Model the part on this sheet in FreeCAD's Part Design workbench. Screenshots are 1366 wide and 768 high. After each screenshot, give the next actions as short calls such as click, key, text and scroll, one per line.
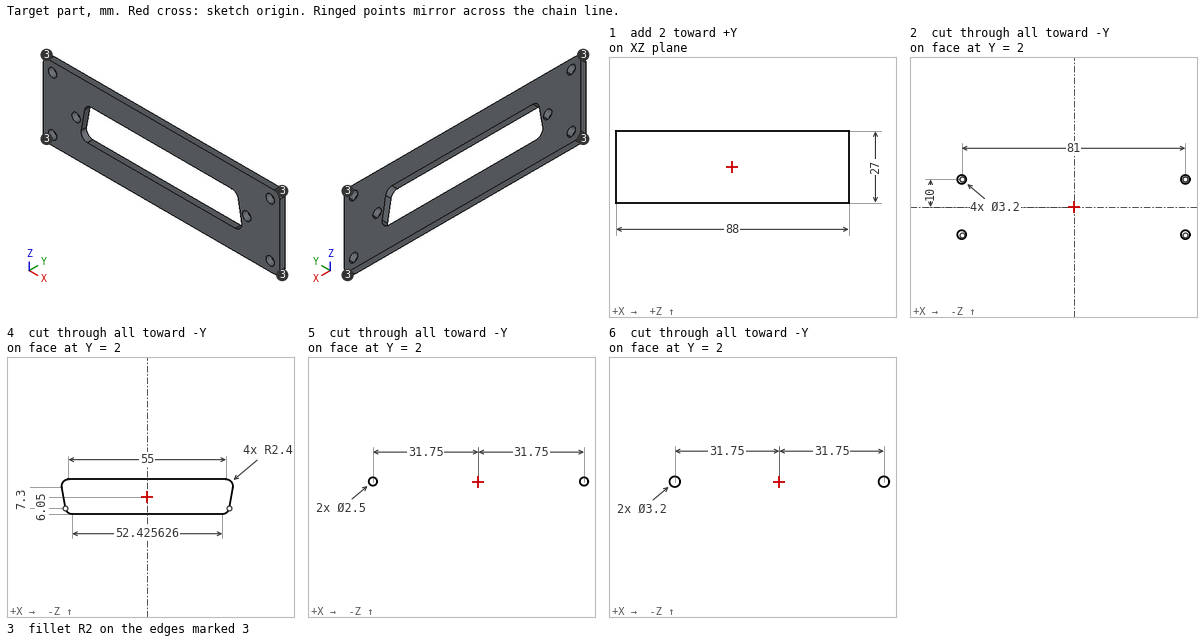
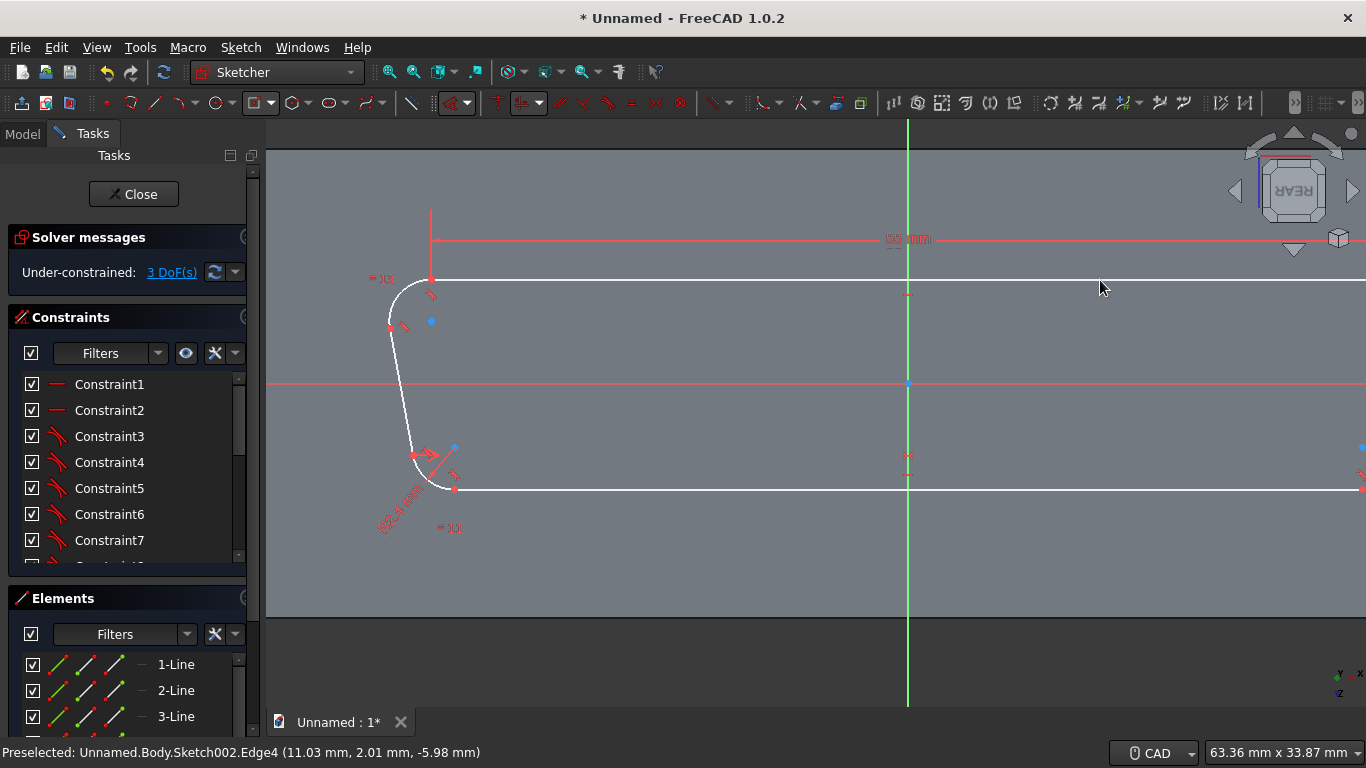
click(397, 367)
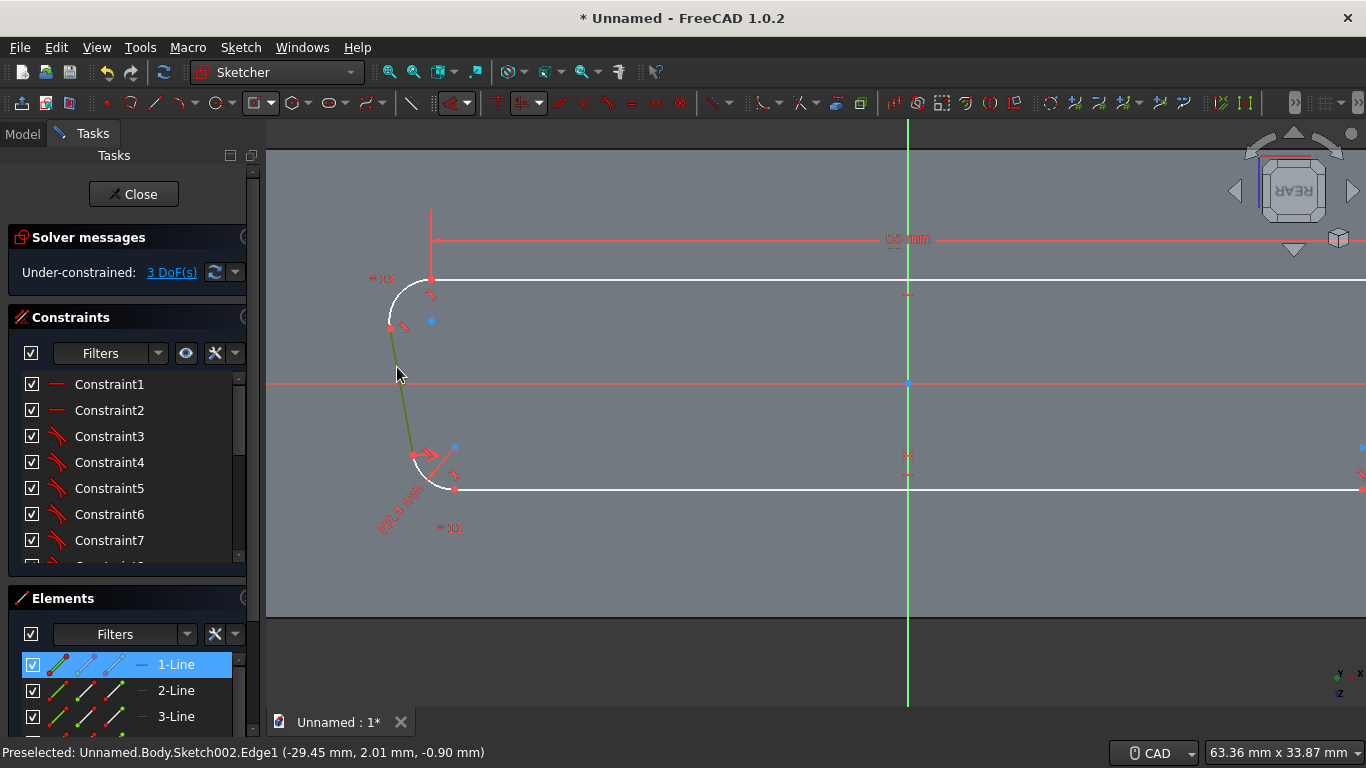
key(i)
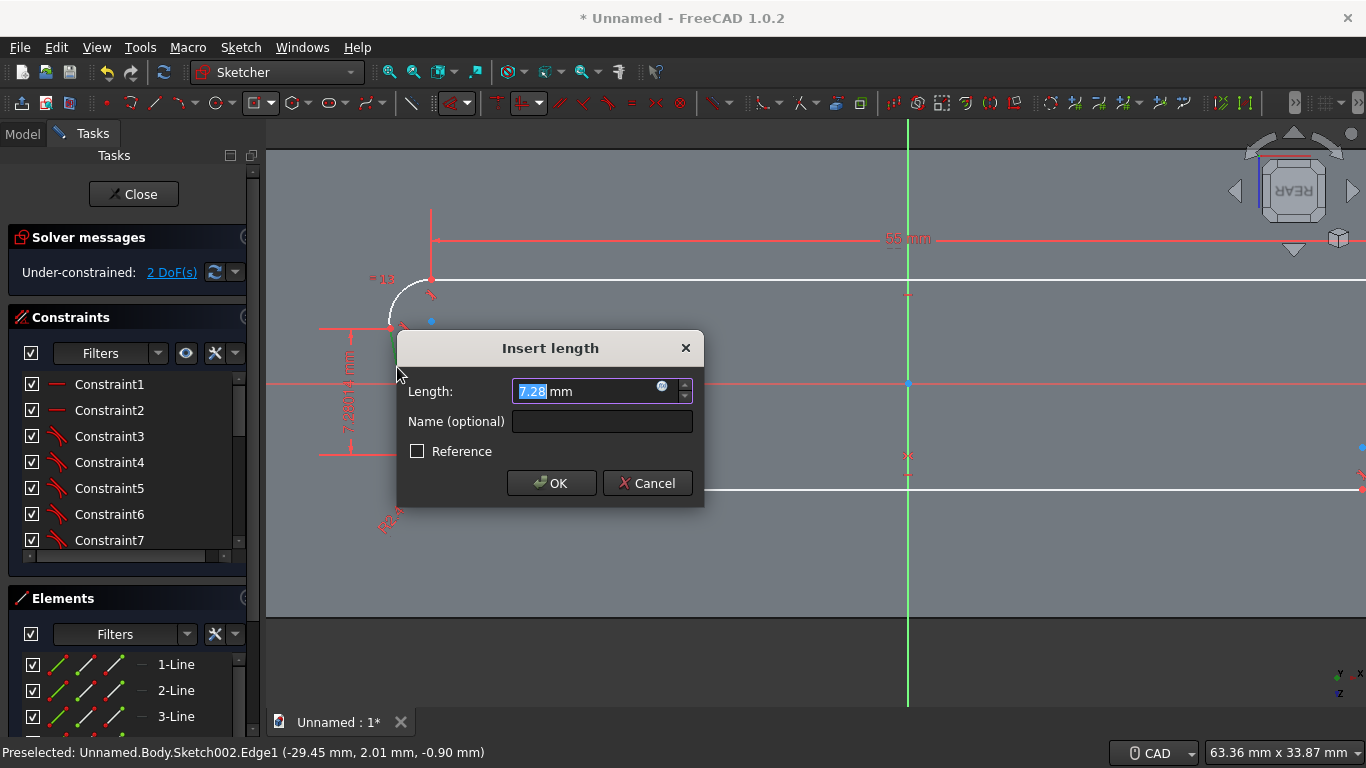
text(7.3)
key(Return)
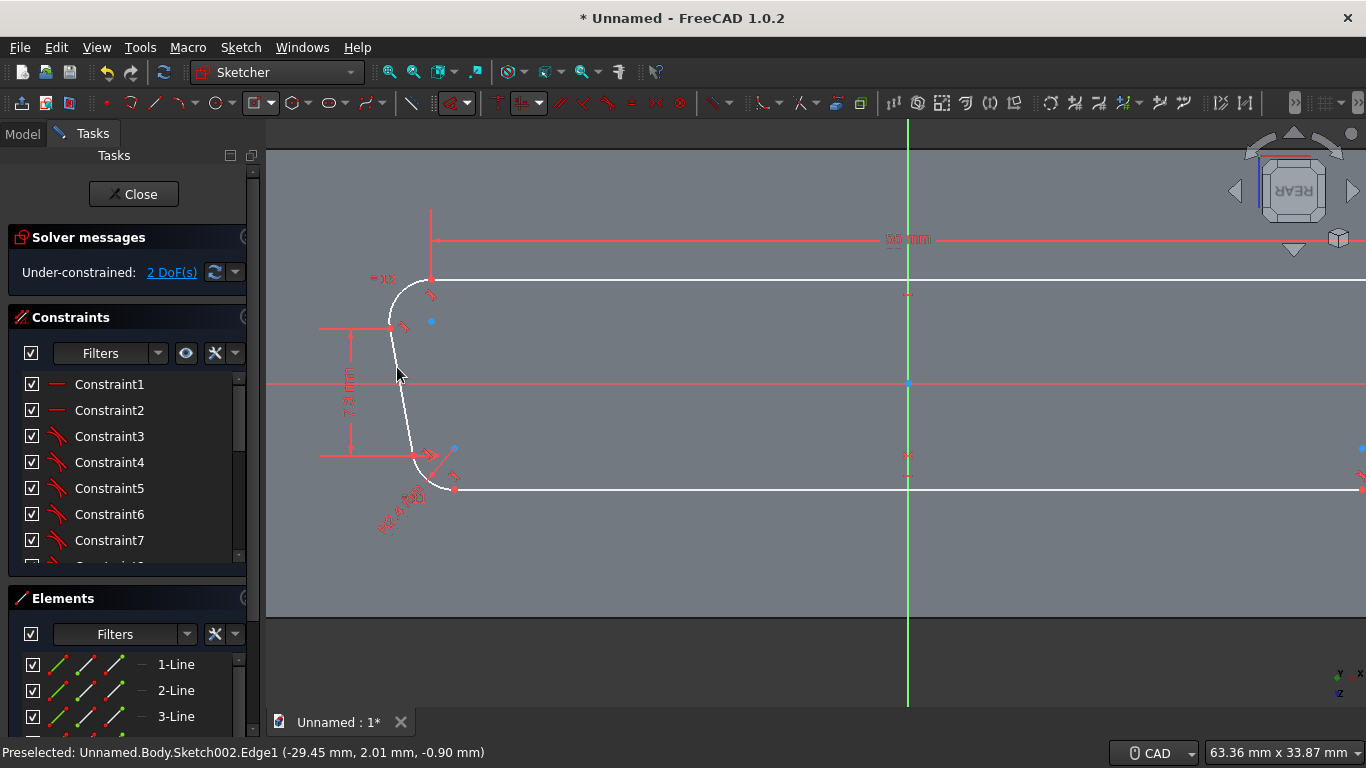
click(454, 490)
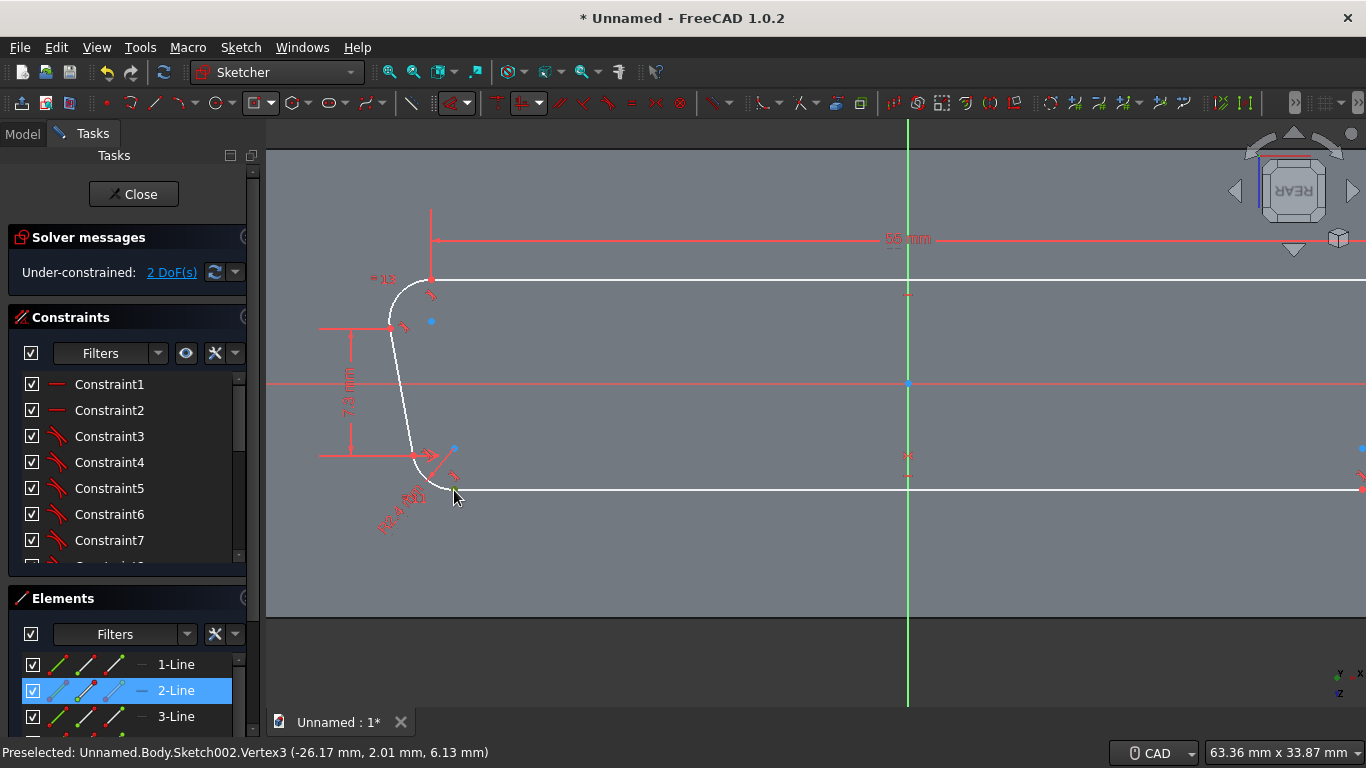
key(i)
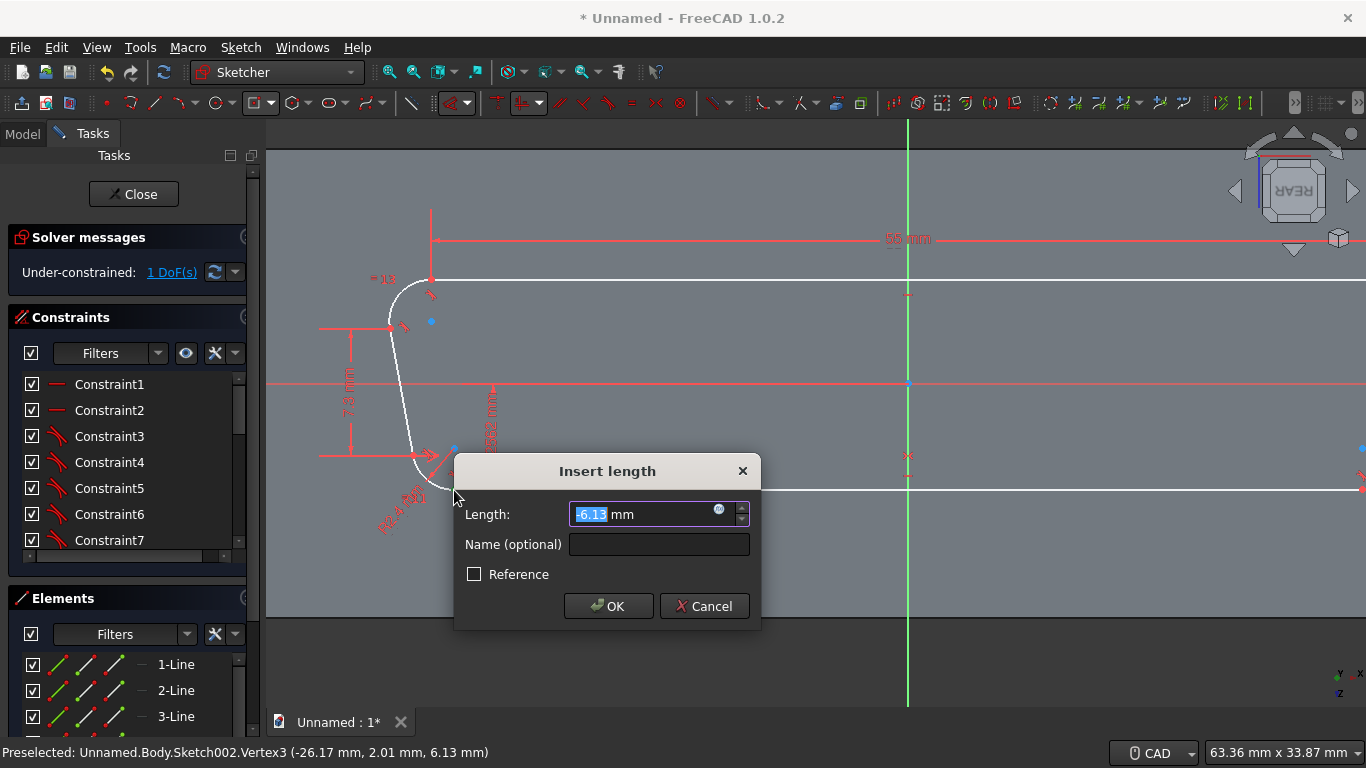
text(-6.05)
key(Return)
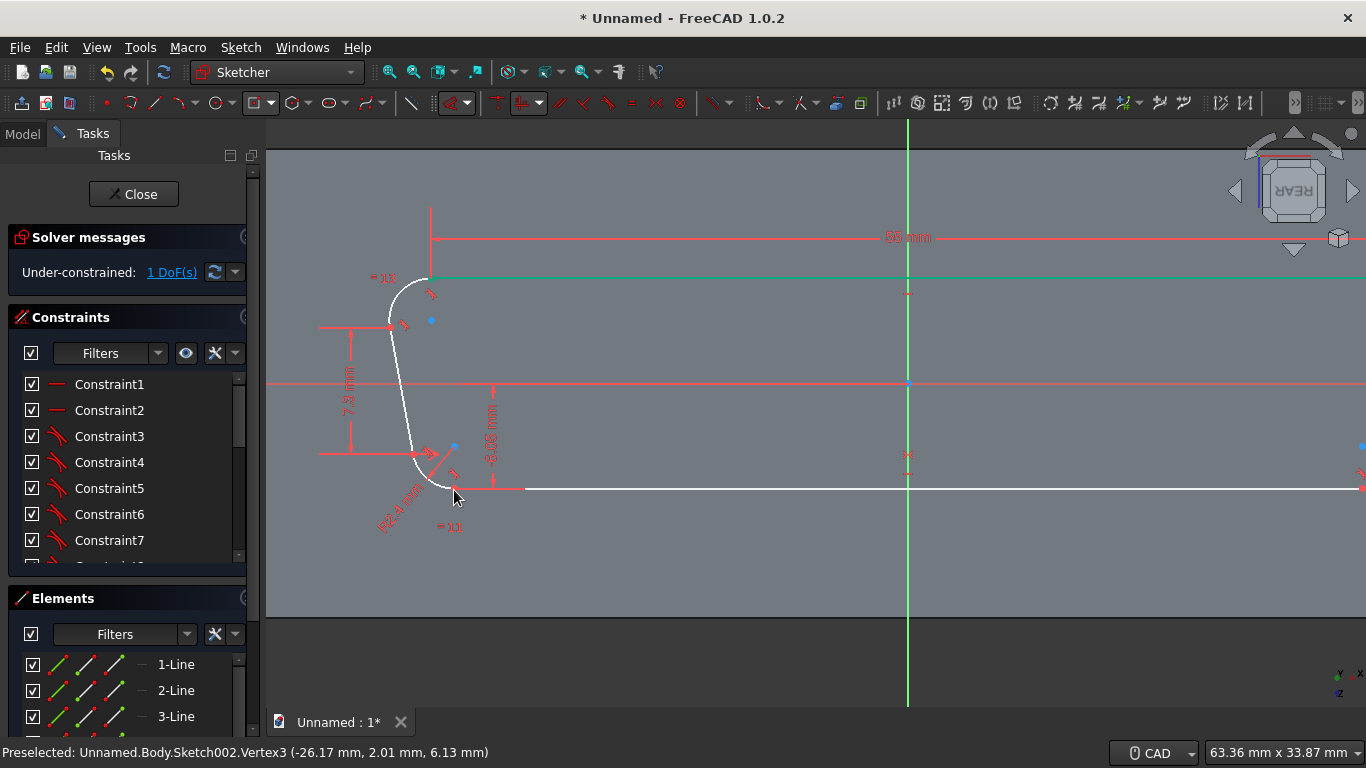
click(727, 489)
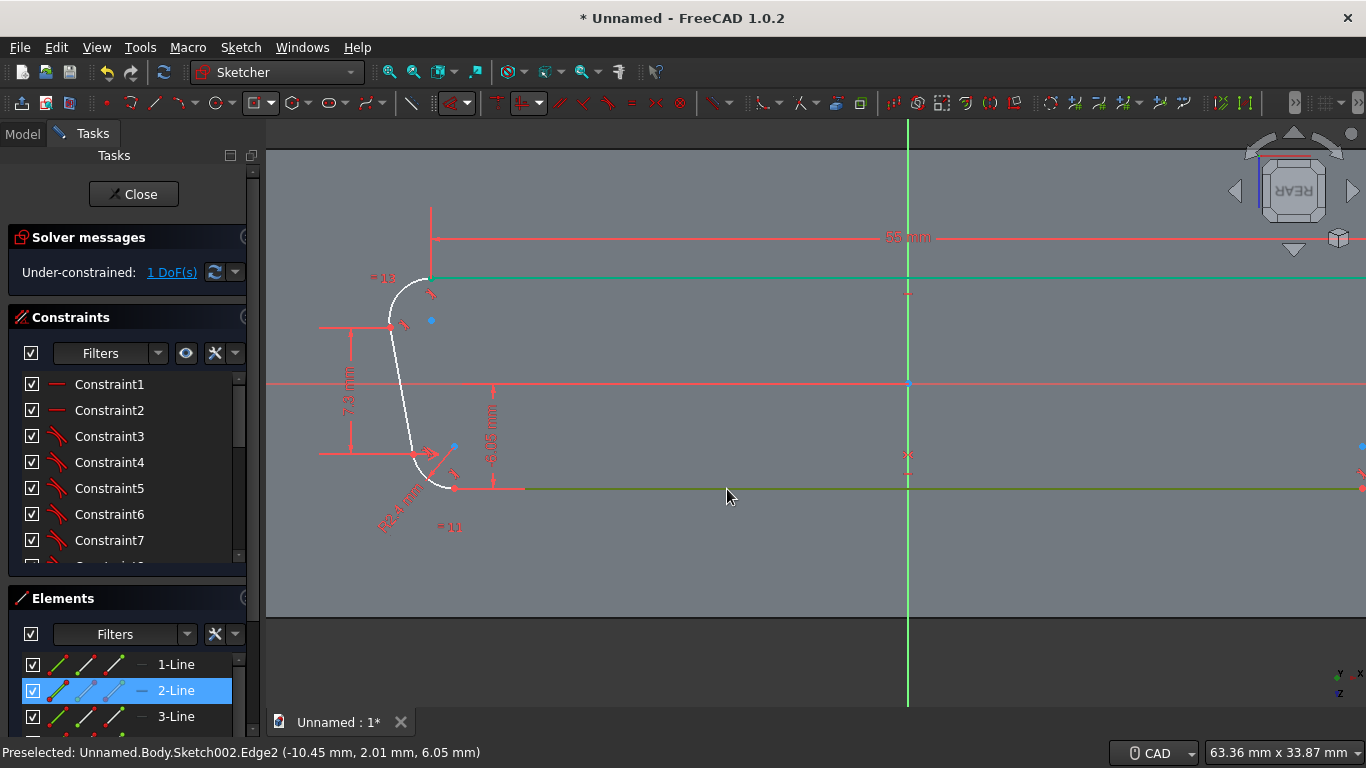
click(470, 104)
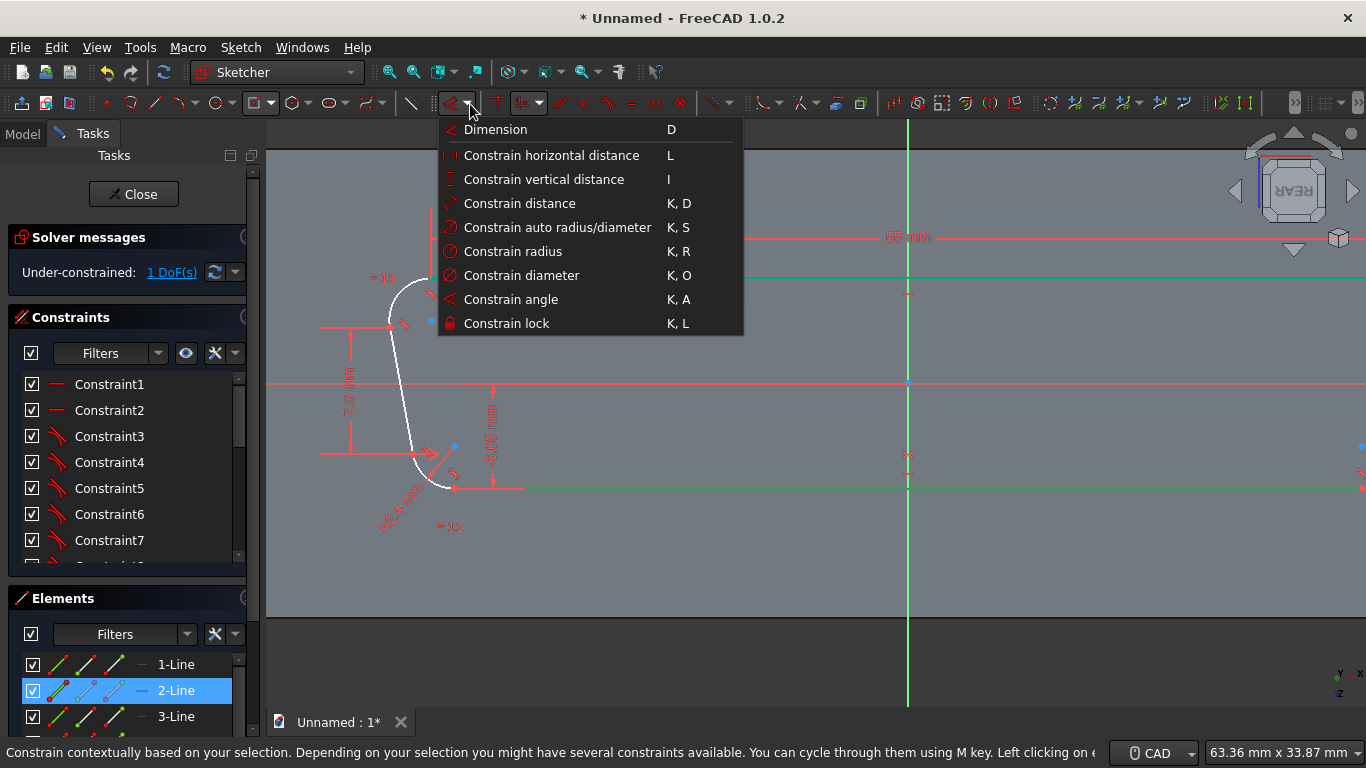
click(591, 155)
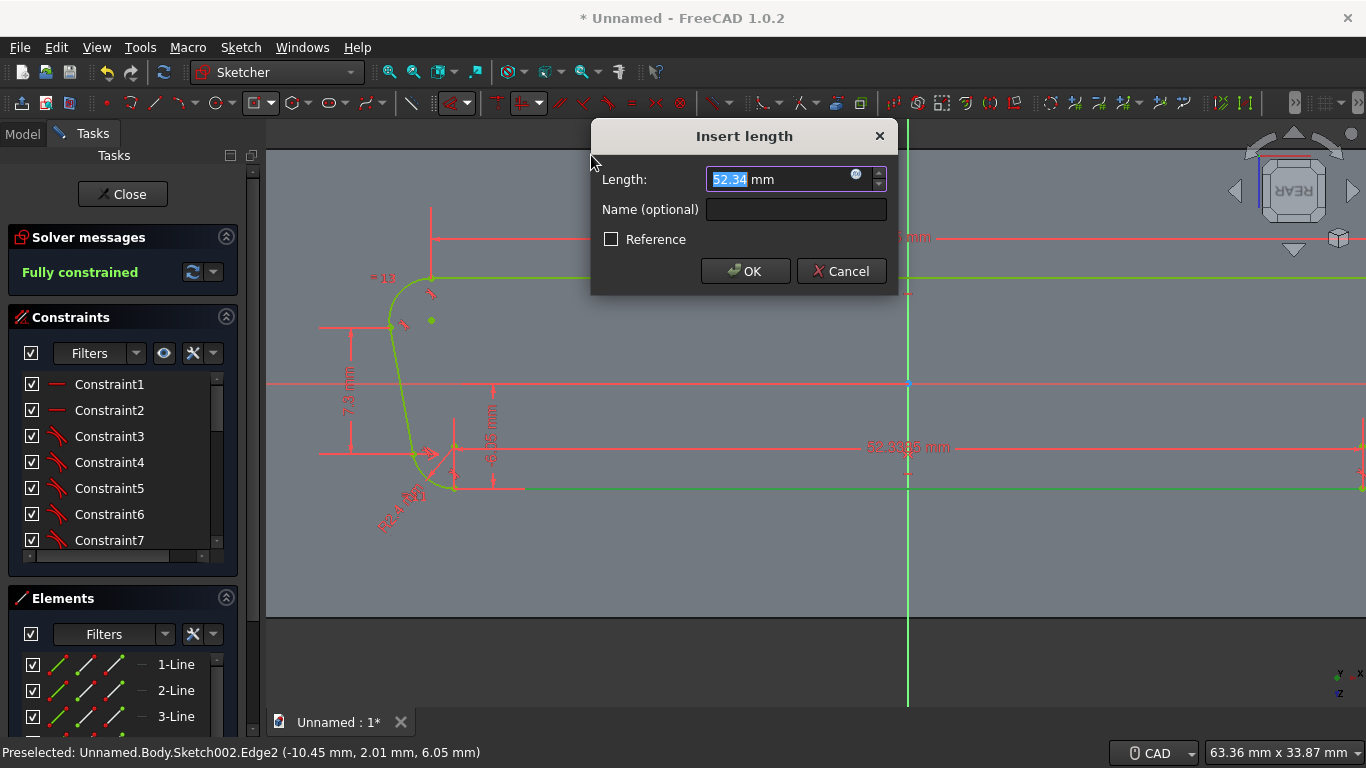
text(52.425626)
key(Return)